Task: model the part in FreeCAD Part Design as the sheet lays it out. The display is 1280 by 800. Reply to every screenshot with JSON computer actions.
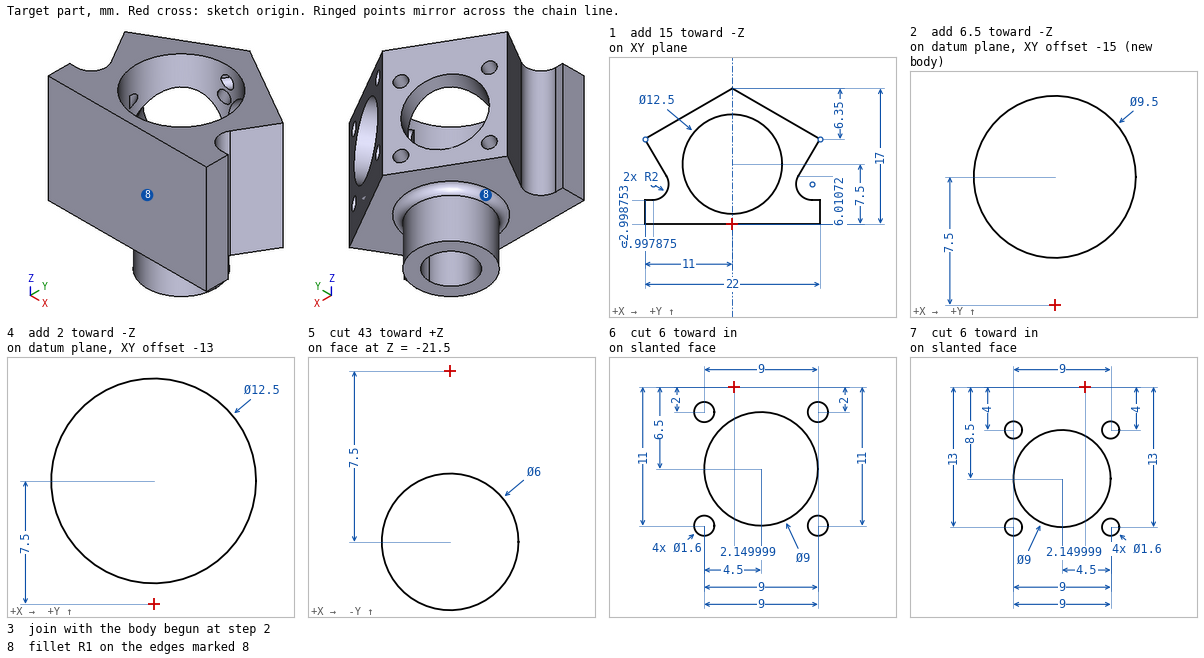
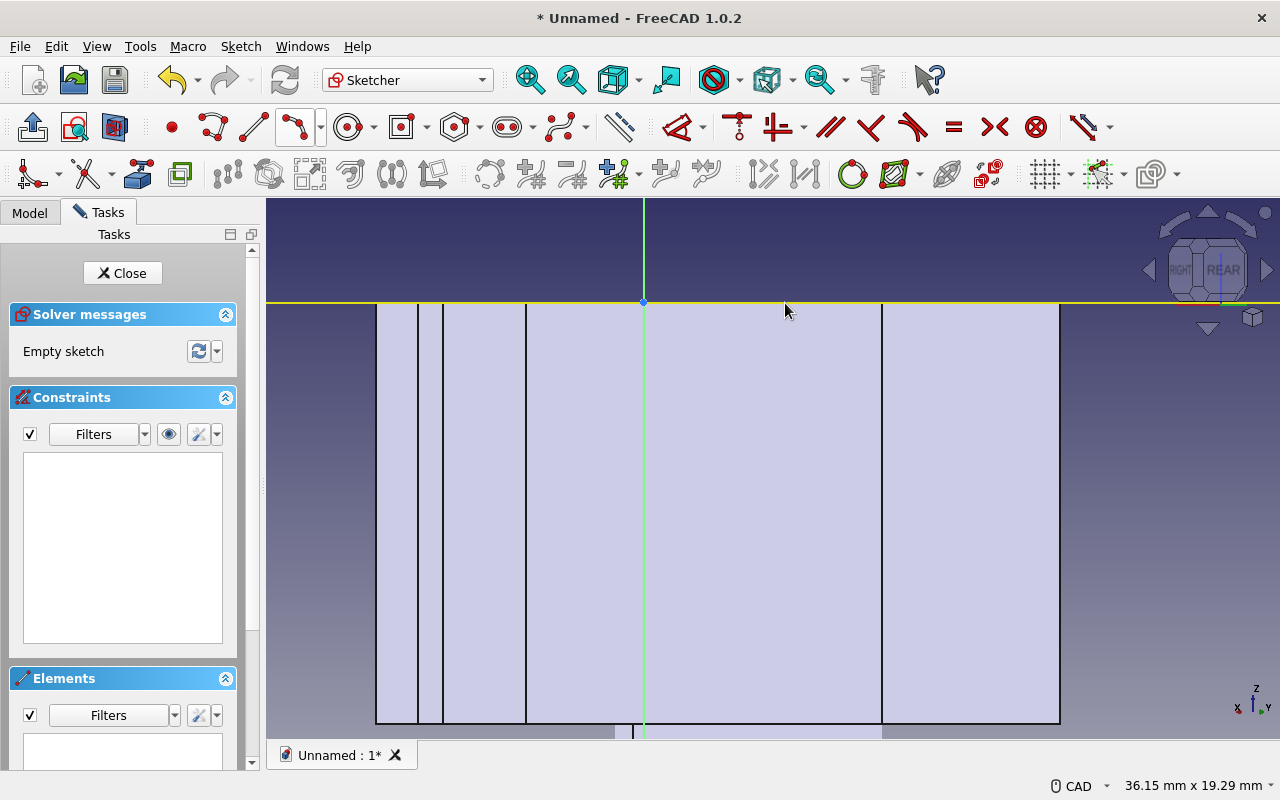
{"action": "left_click", "coordinate": [348, 128]}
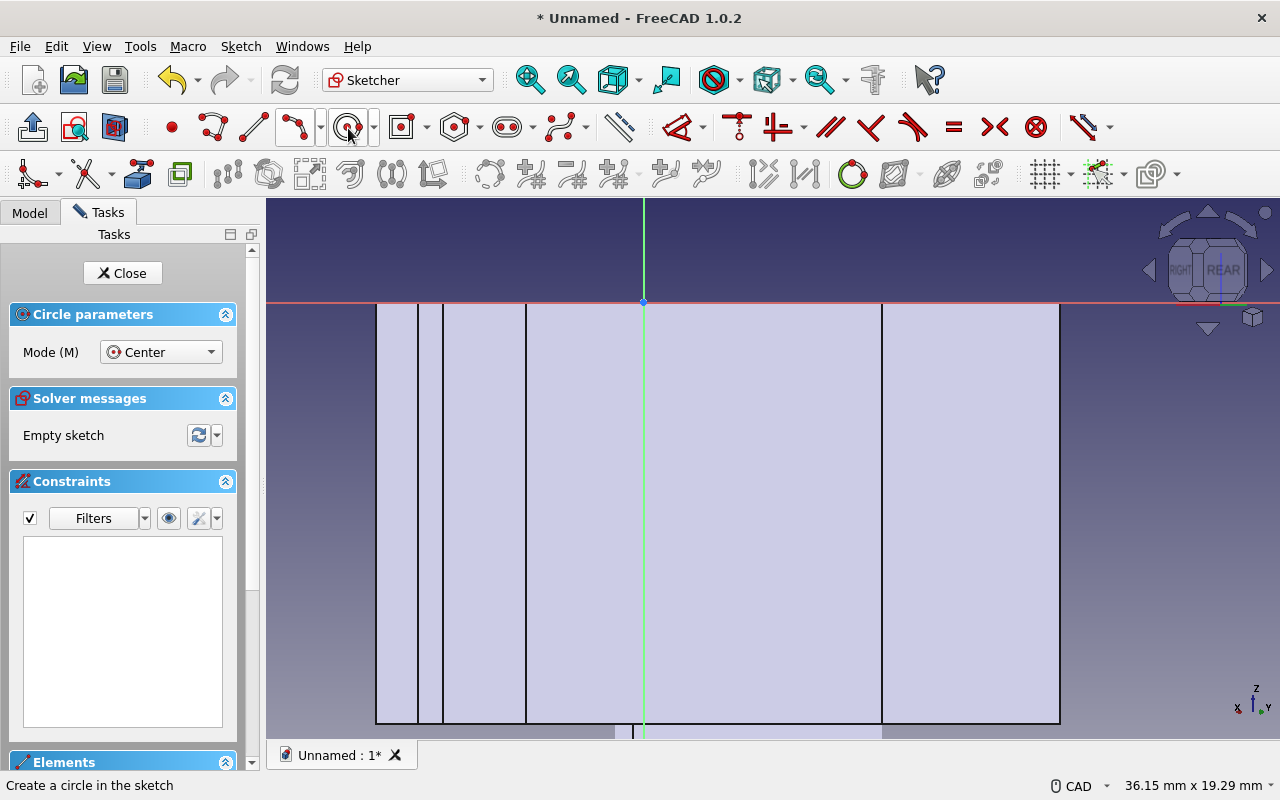
{"action": "left_click", "coordinate": [704, 485]}
{"action": "mouse_move", "coordinate": [793, 396]}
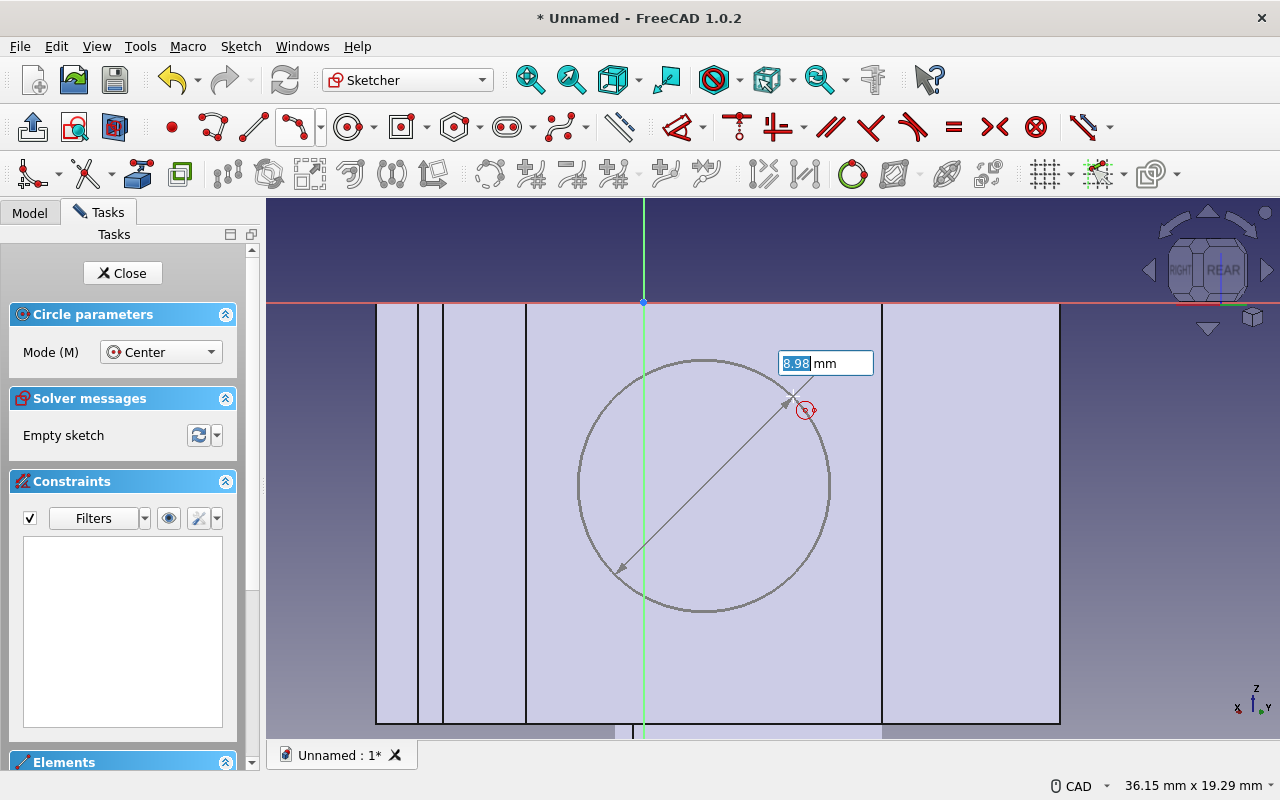
{"action": "type", "text": "9"}
{"action": "key", "text": "Return"}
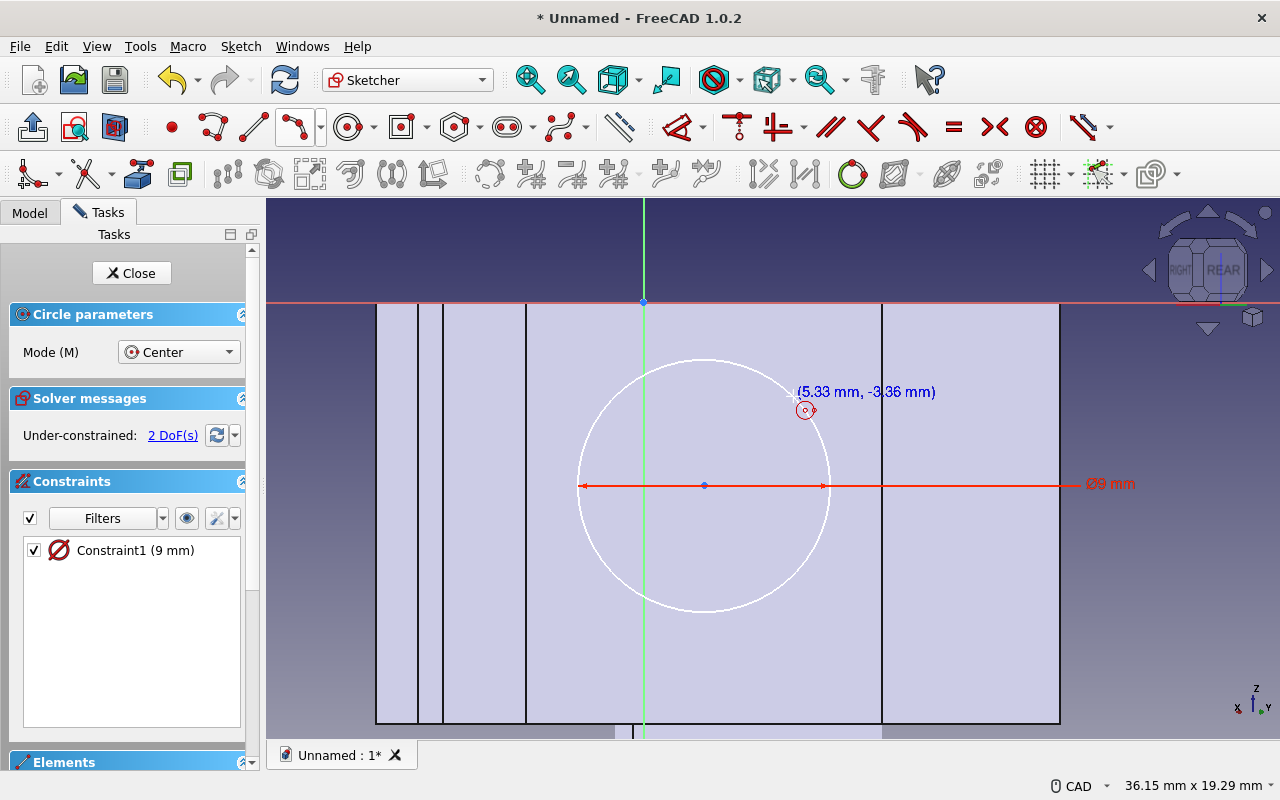
{"action": "left_click", "coordinate": [578, 611]}
{"action": "mouse_move", "coordinate": [593, 596]}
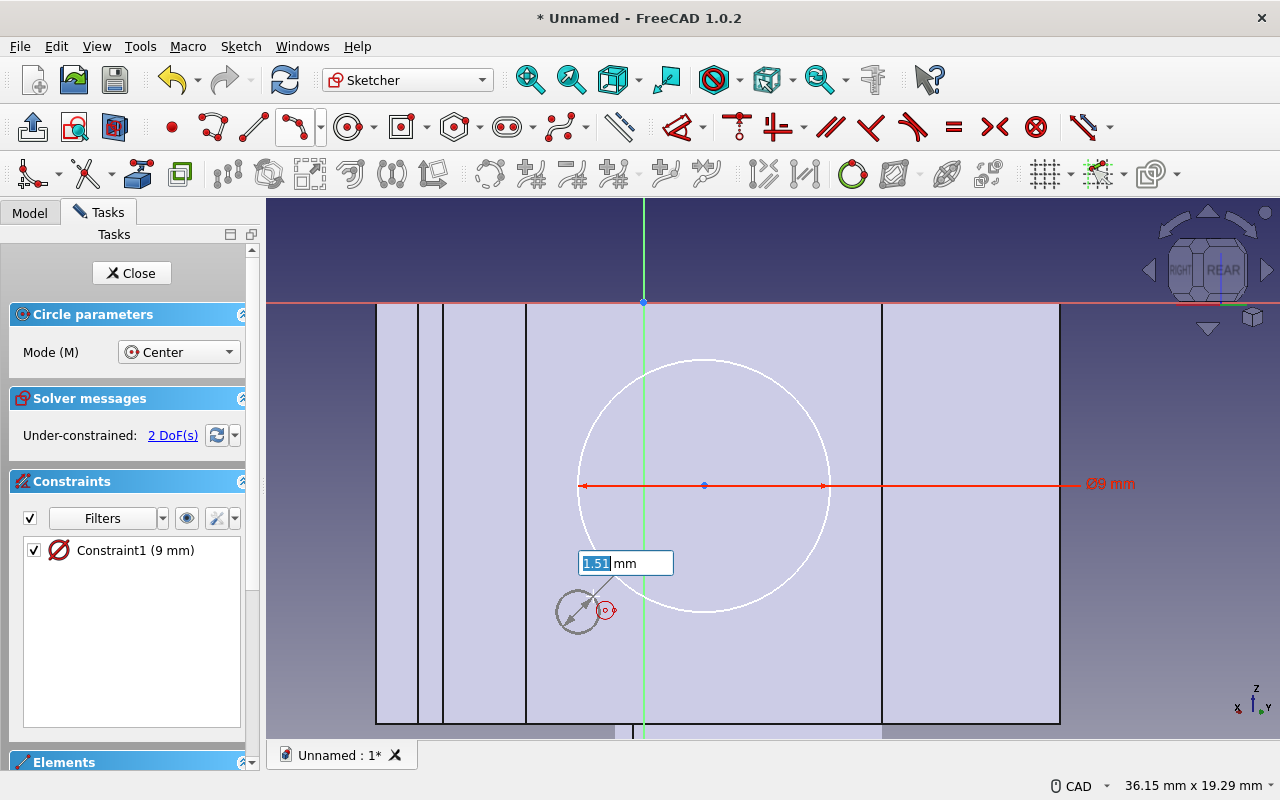
{"action": "type", "text": "1.6"}
{"action": "key", "text": "Return"}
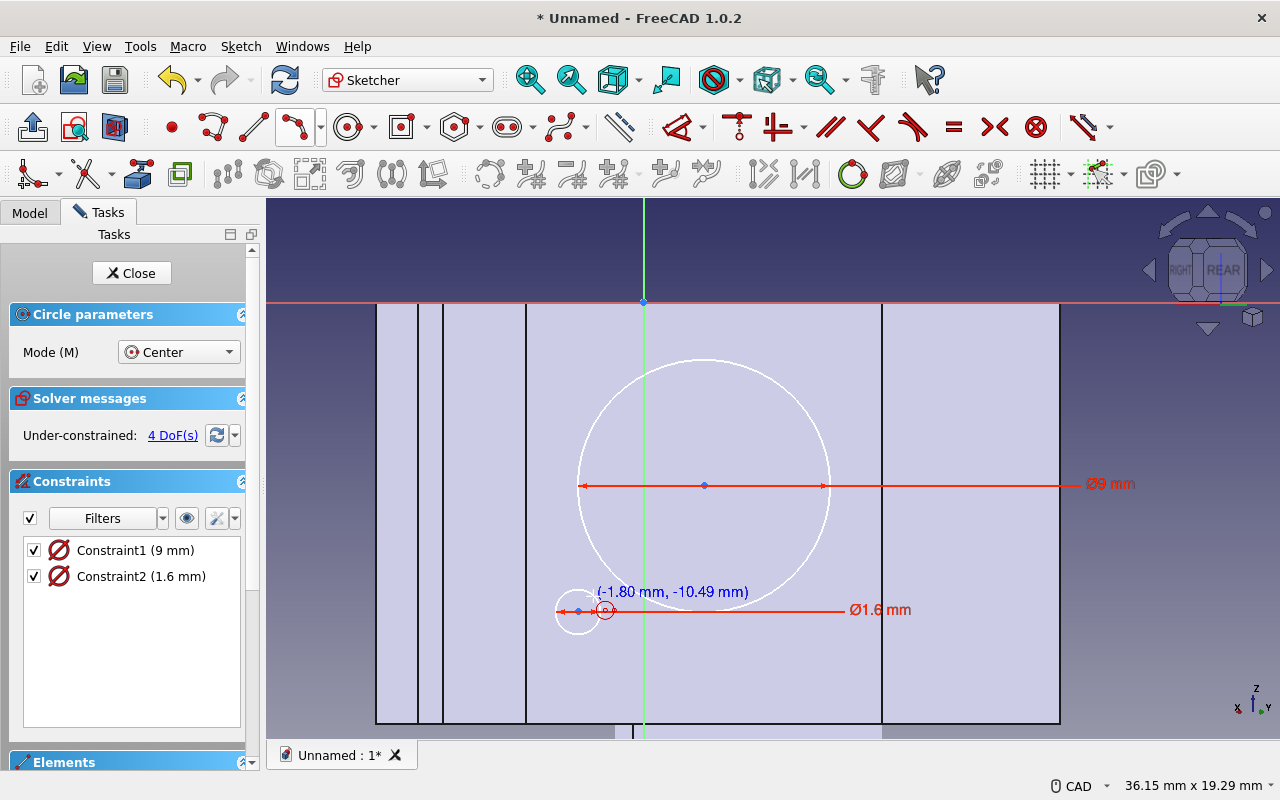
{"action": "left_click", "coordinate": [578, 359]}
{"action": "mouse_move", "coordinate": [593, 343]}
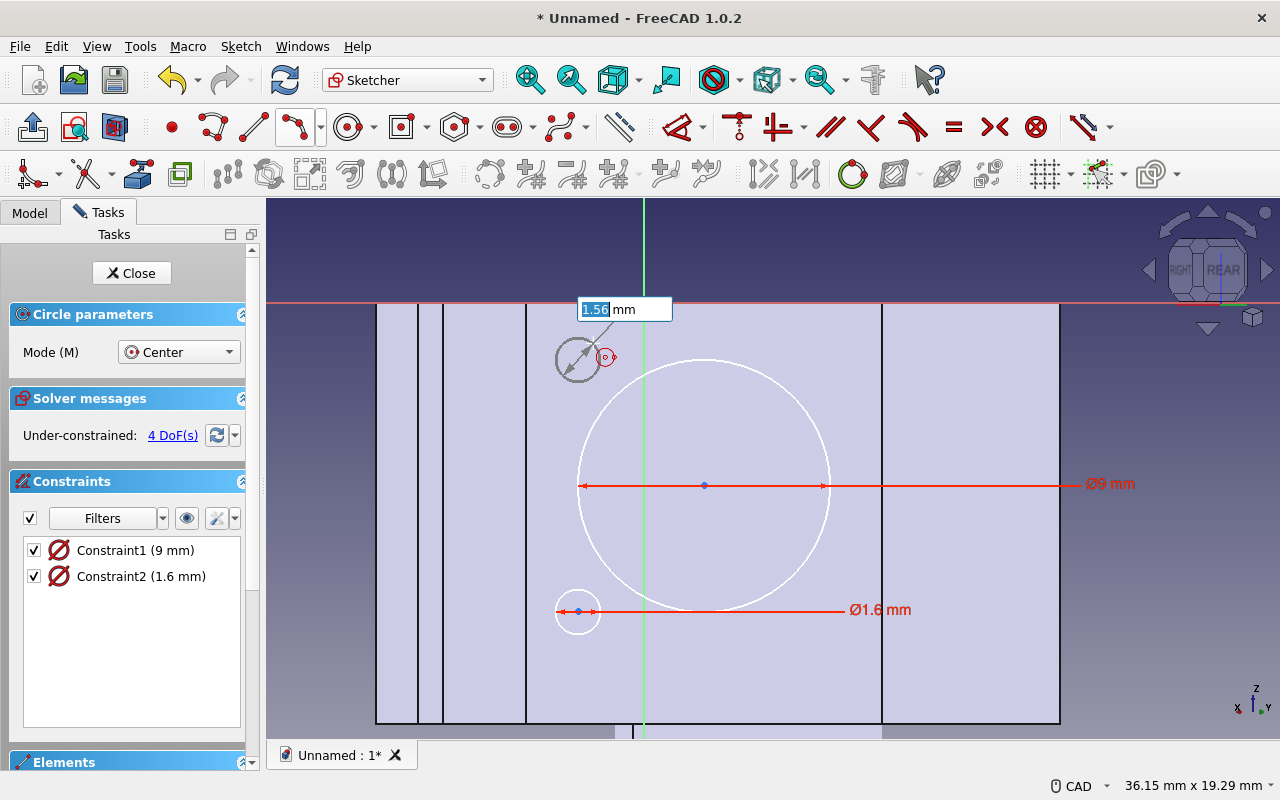
{"action": "type", "text": "1.6"}
{"action": "key", "text": "Return"}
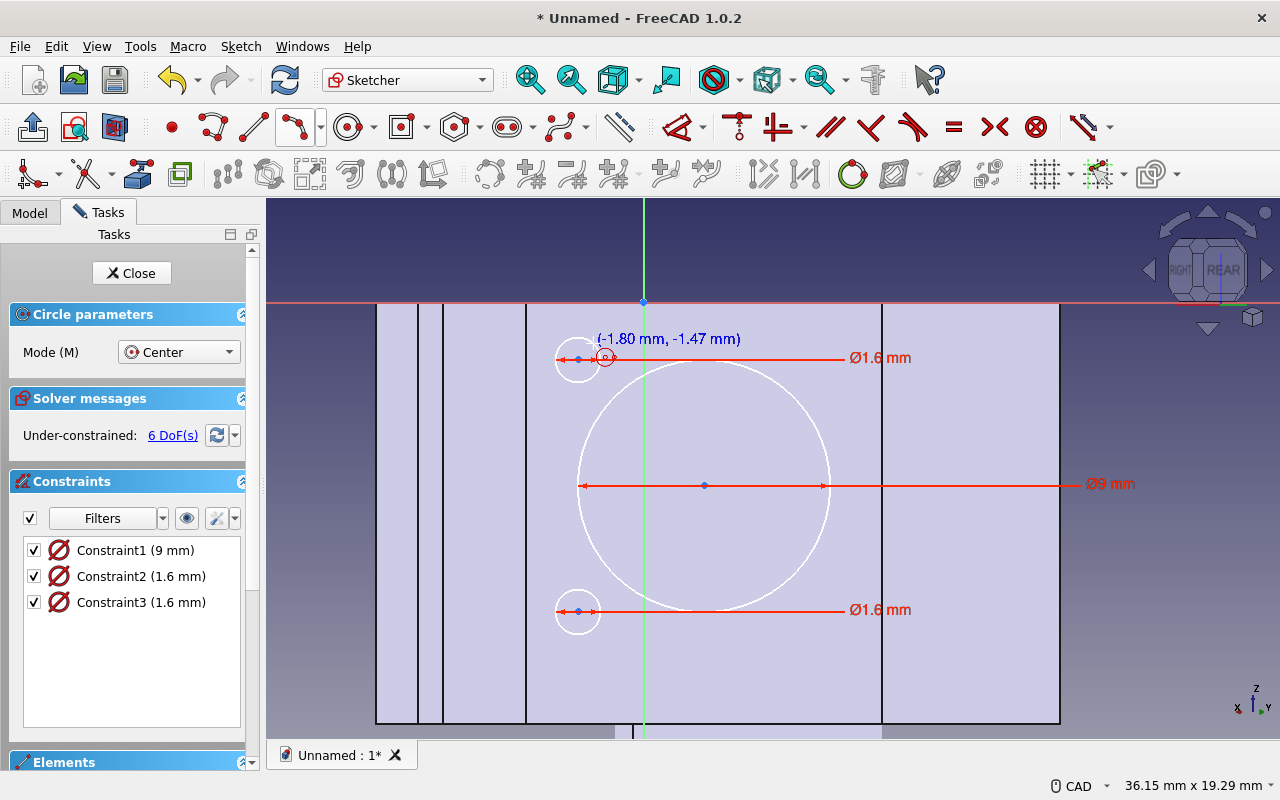
{"action": "left_click", "coordinate": [830, 359]}
{"action": "mouse_move", "coordinate": [846, 343]}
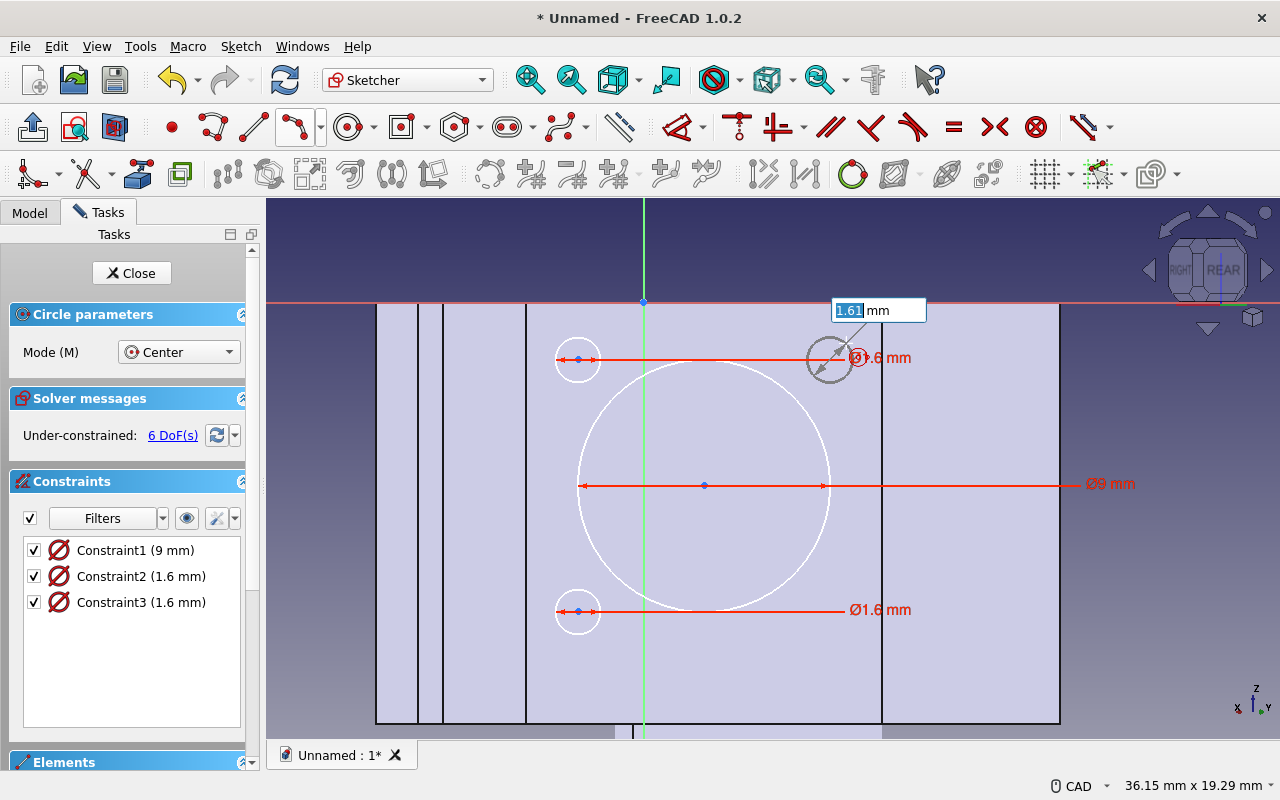
{"action": "type", "text": "1.6"}
{"action": "key", "text": "Return"}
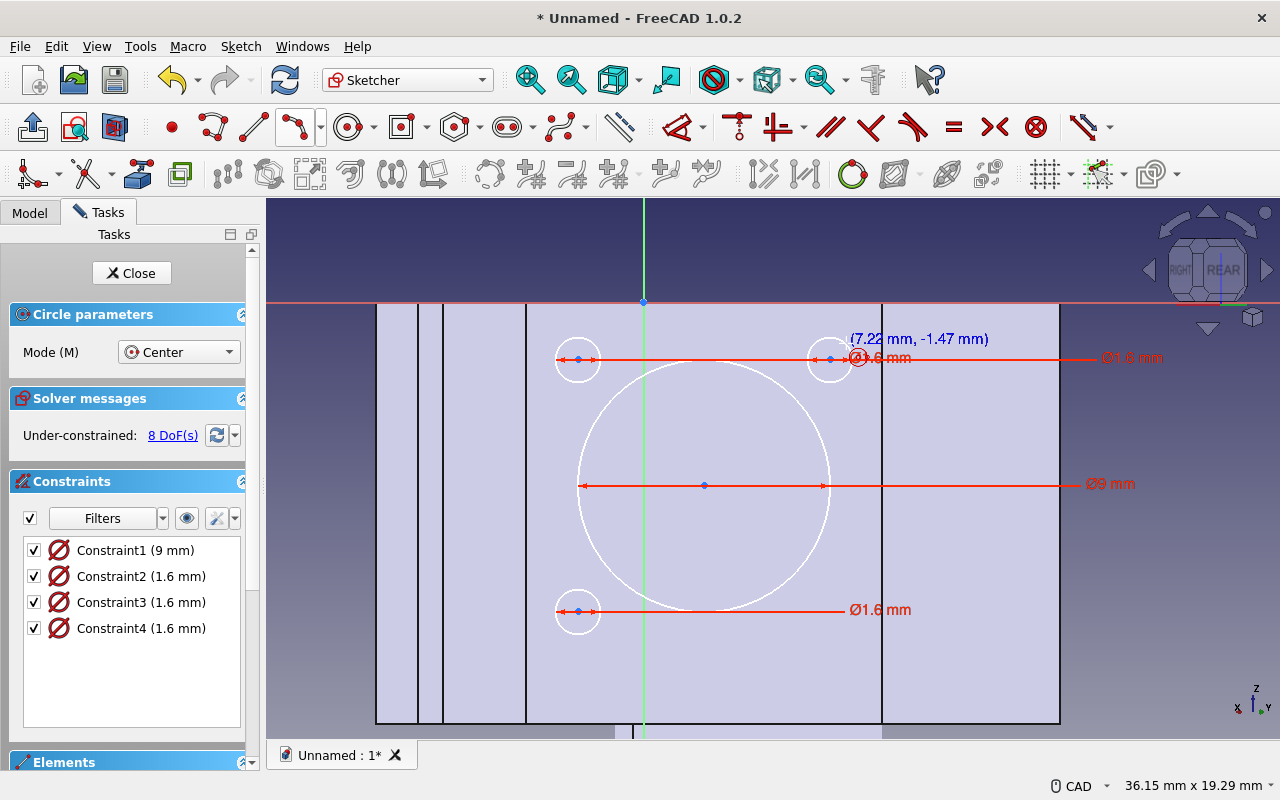
{"action": "left_click", "coordinate": [830, 611]}
{"action": "mouse_move", "coordinate": [846, 596]}